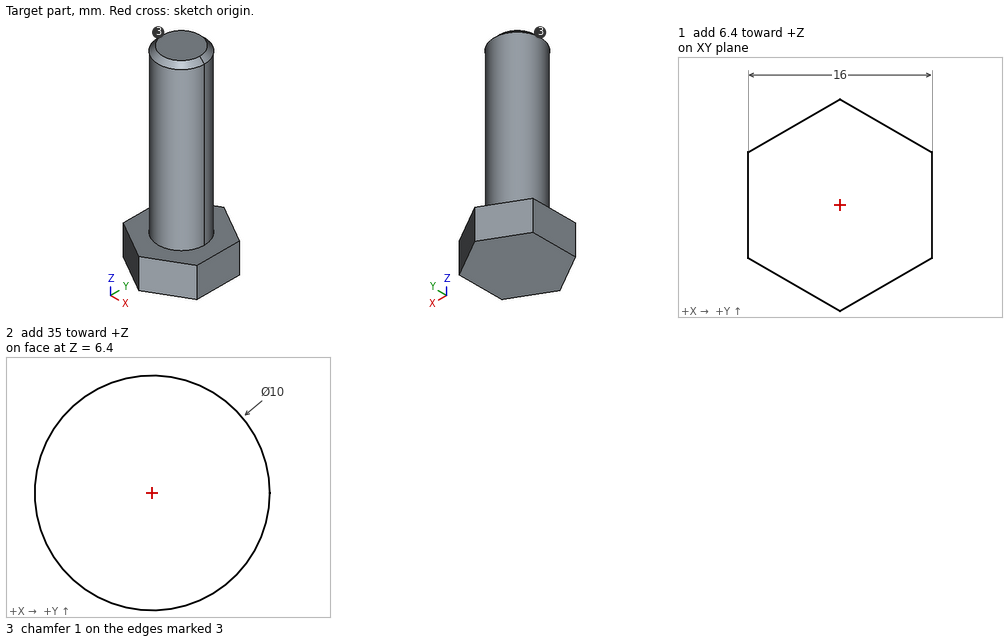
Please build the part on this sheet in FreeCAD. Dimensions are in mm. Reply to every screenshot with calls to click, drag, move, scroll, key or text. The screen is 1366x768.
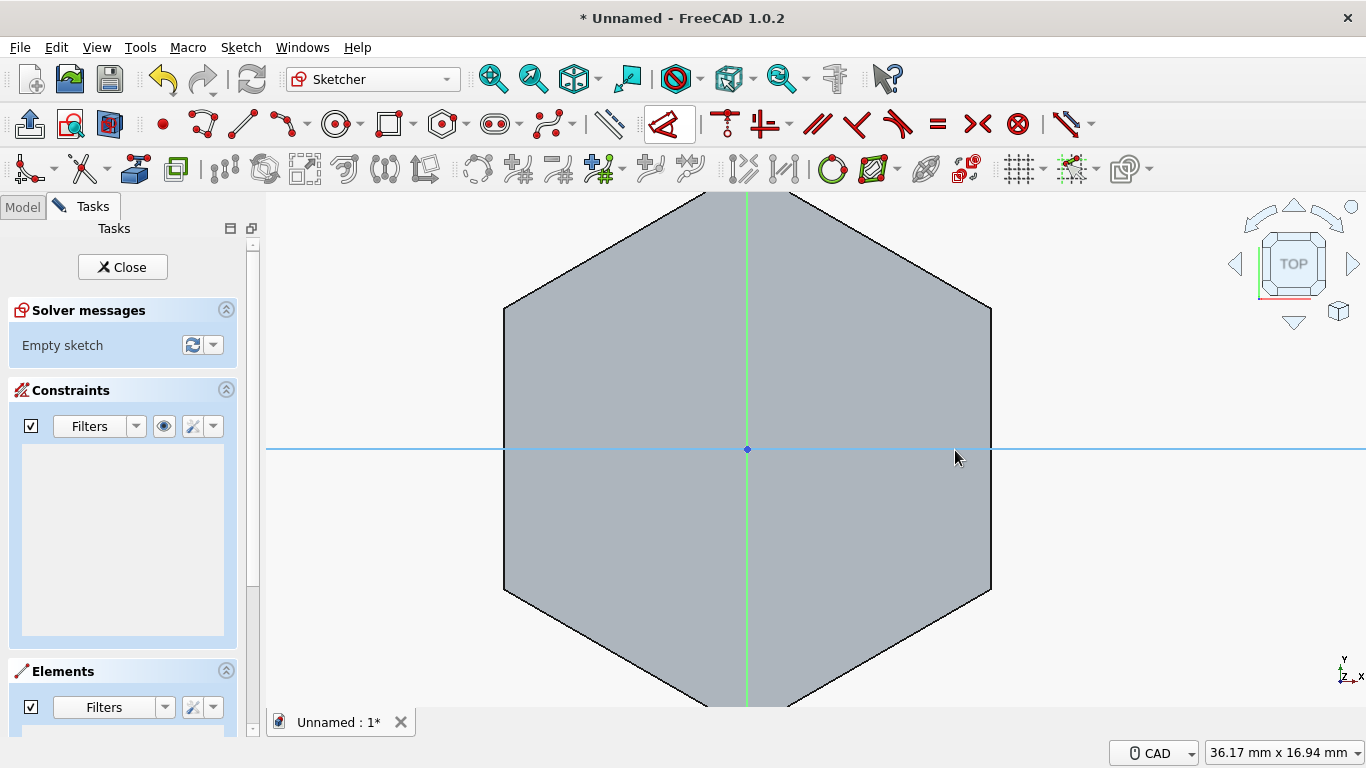
click(336, 124)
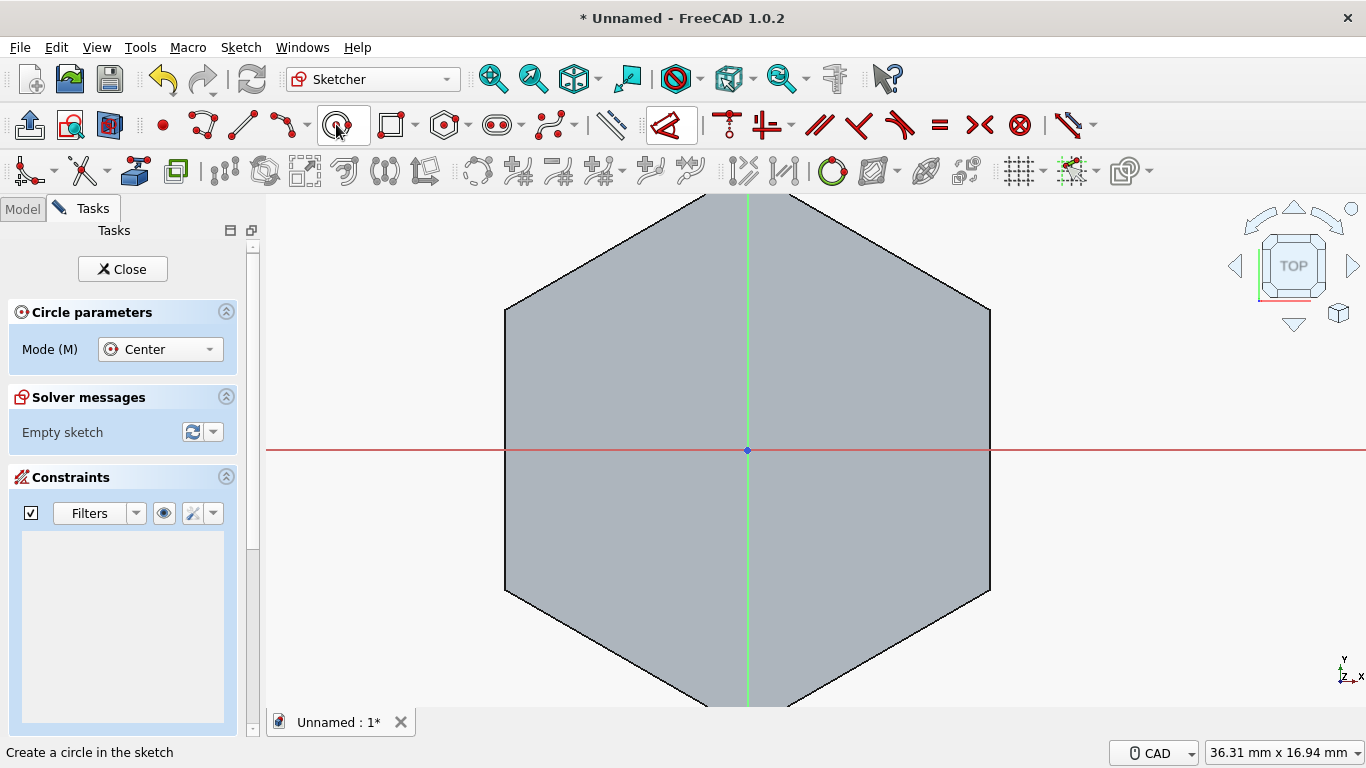
click(748, 450)
click(855, 343)
key(Escape)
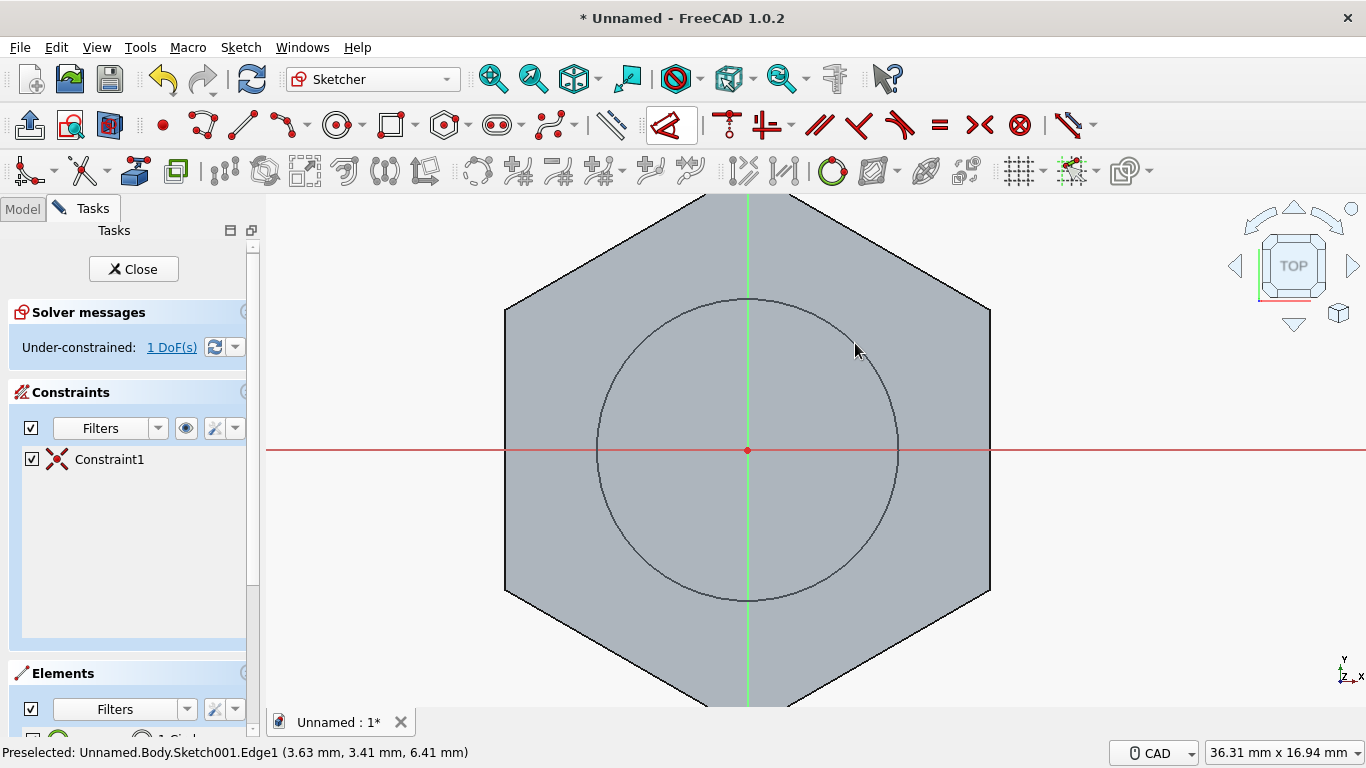
click(666, 126)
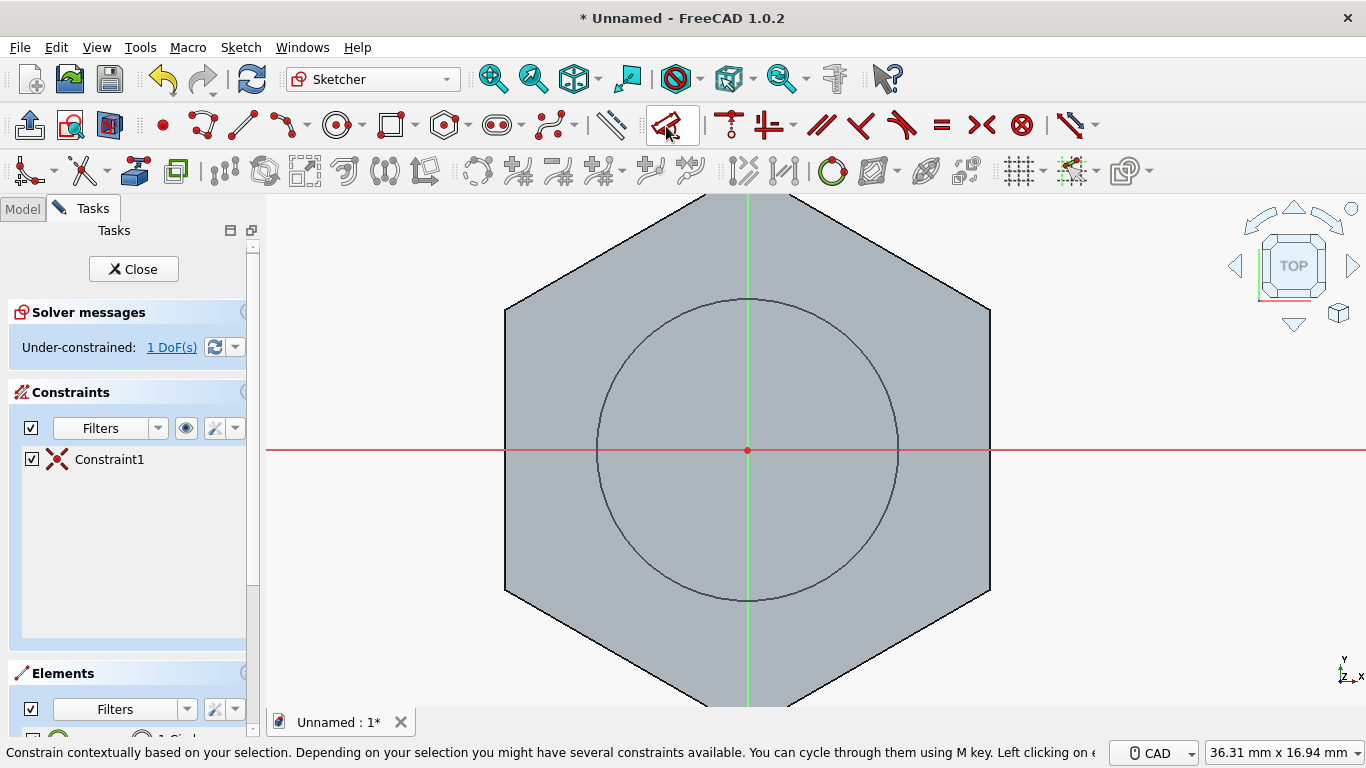
click(854, 343)
click(877, 320)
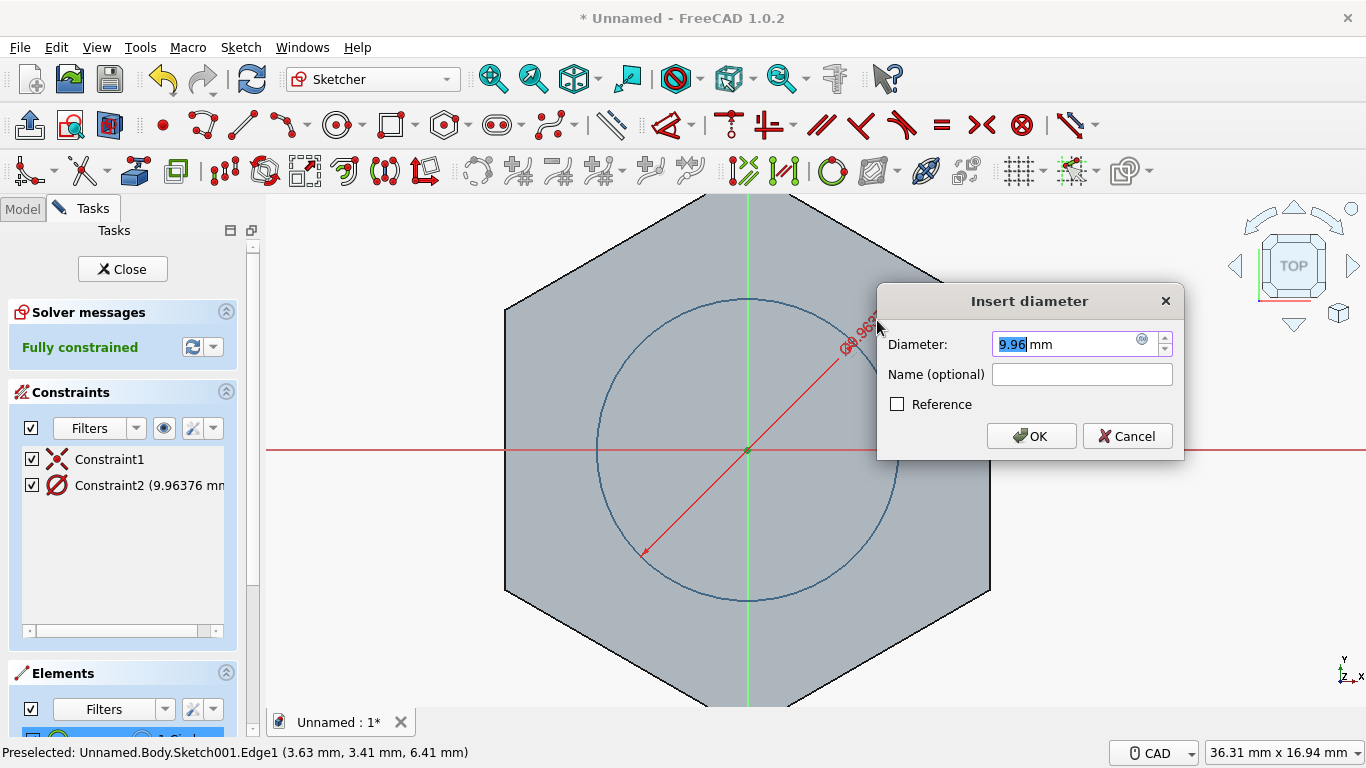
text(10)
key(Return)
key(Escape)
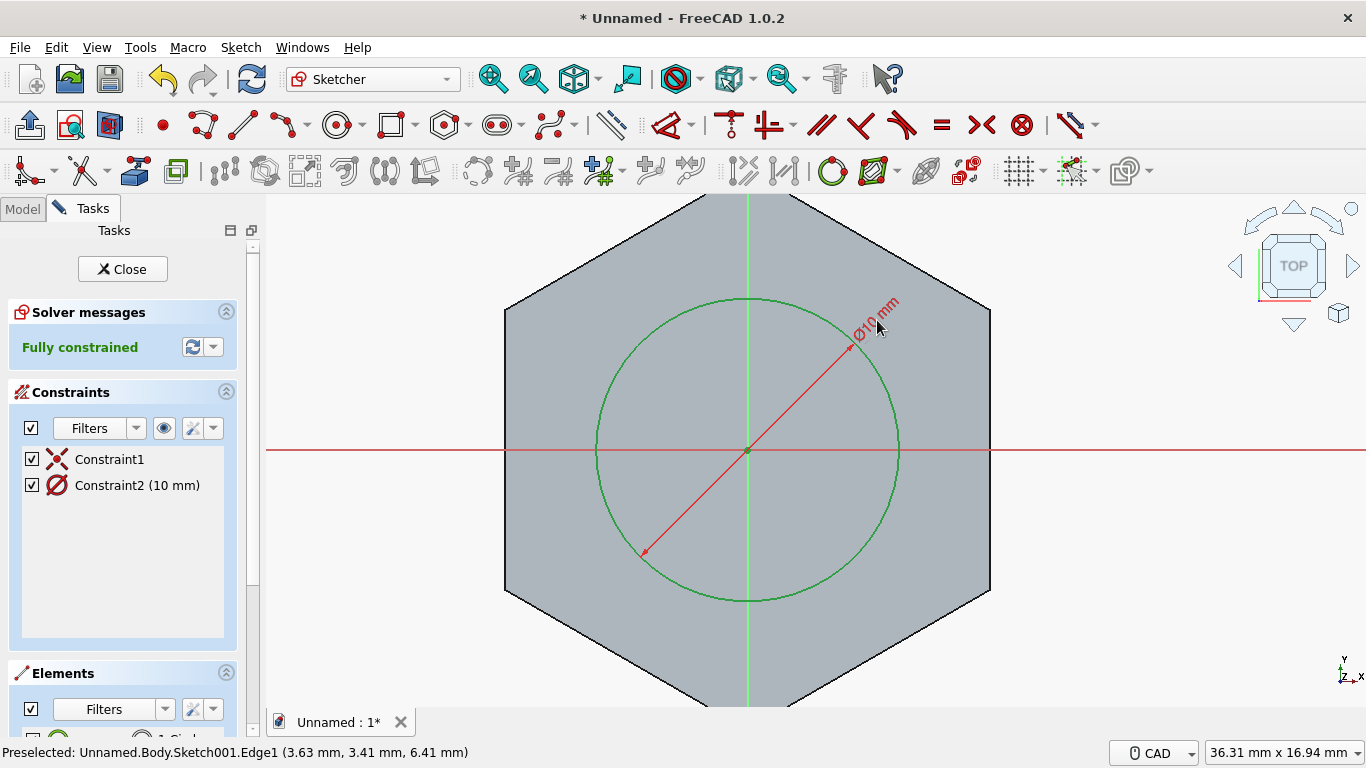
click(123, 269)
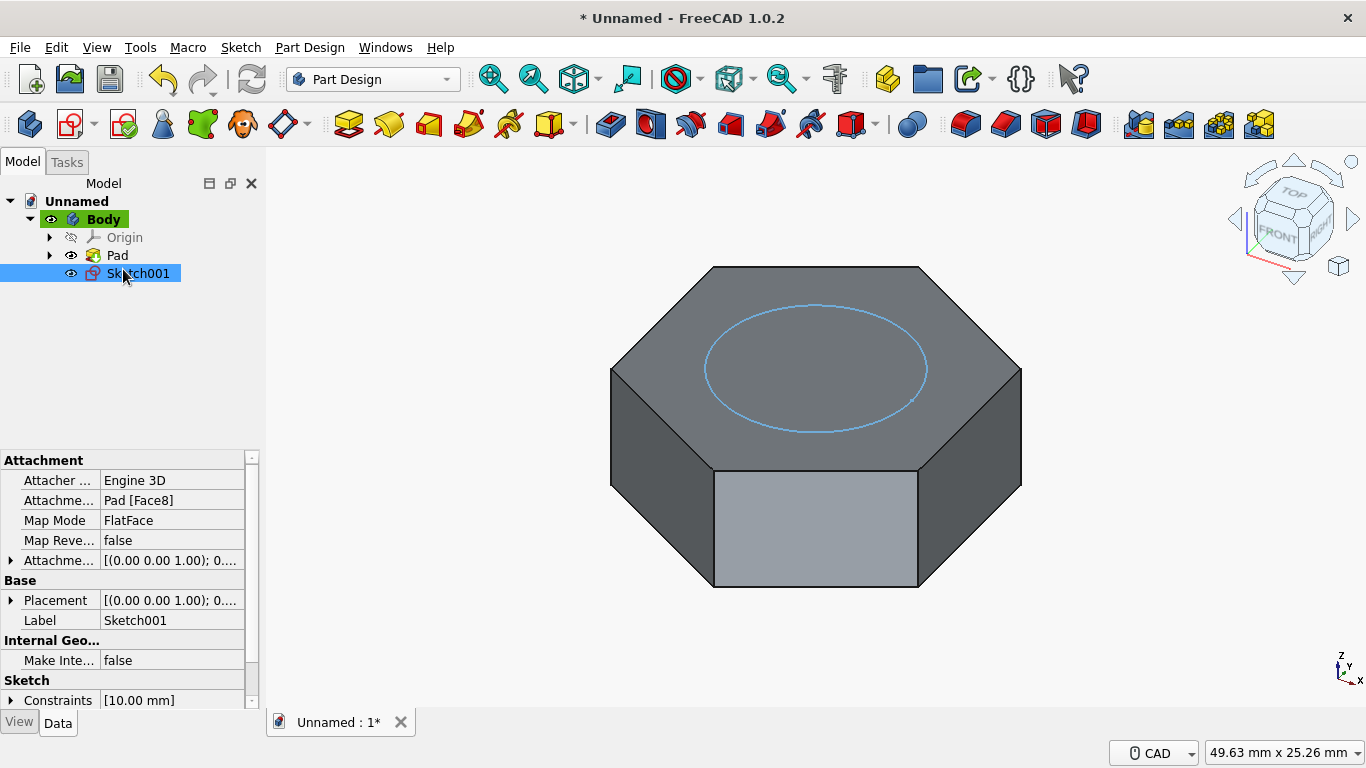
click(350, 124)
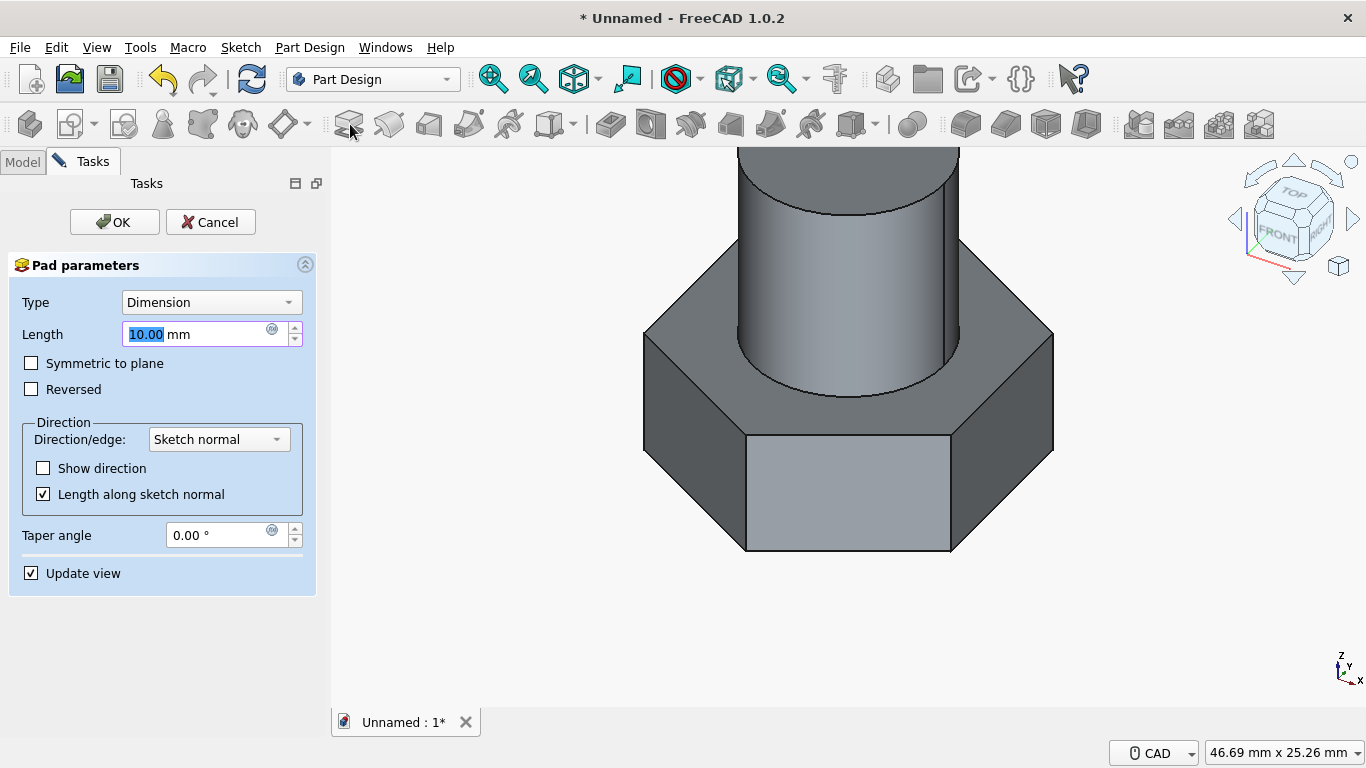
text(35)
key(Tab)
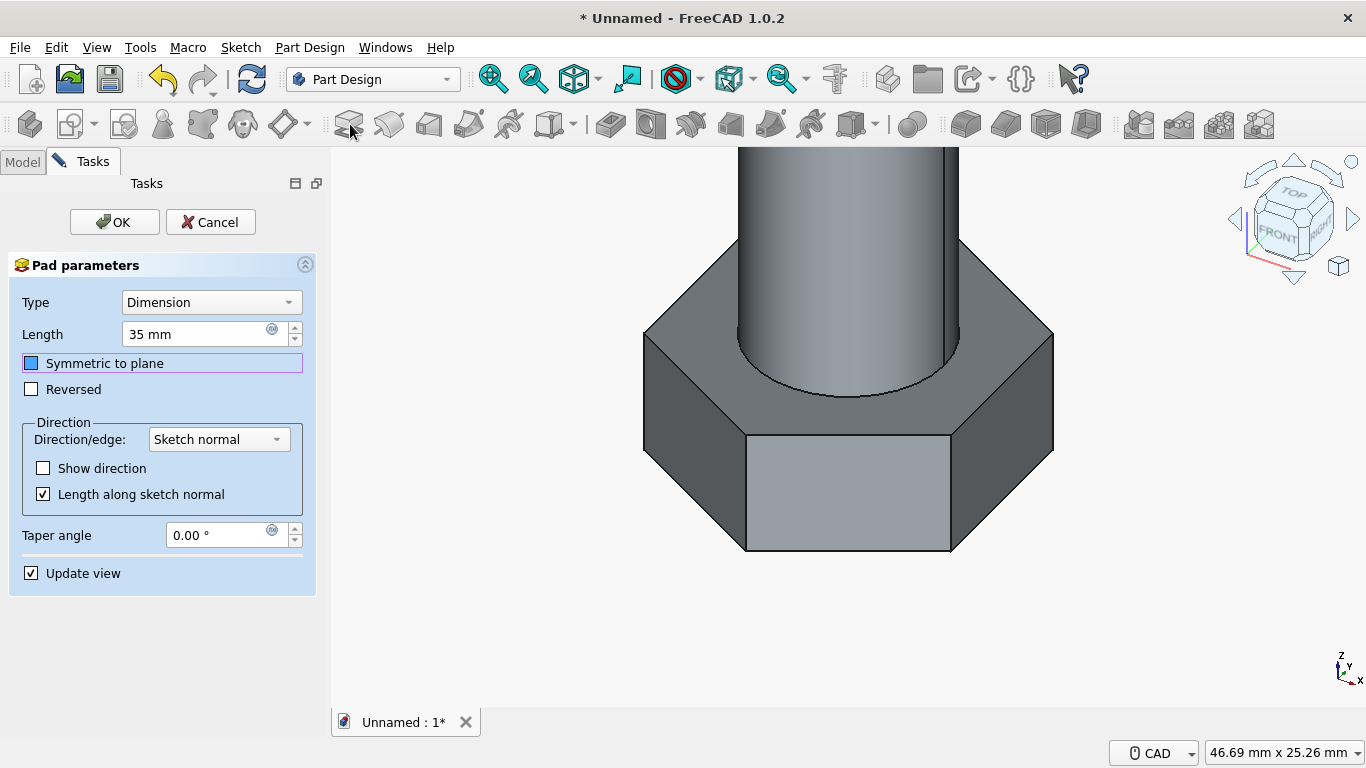
click(115, 222)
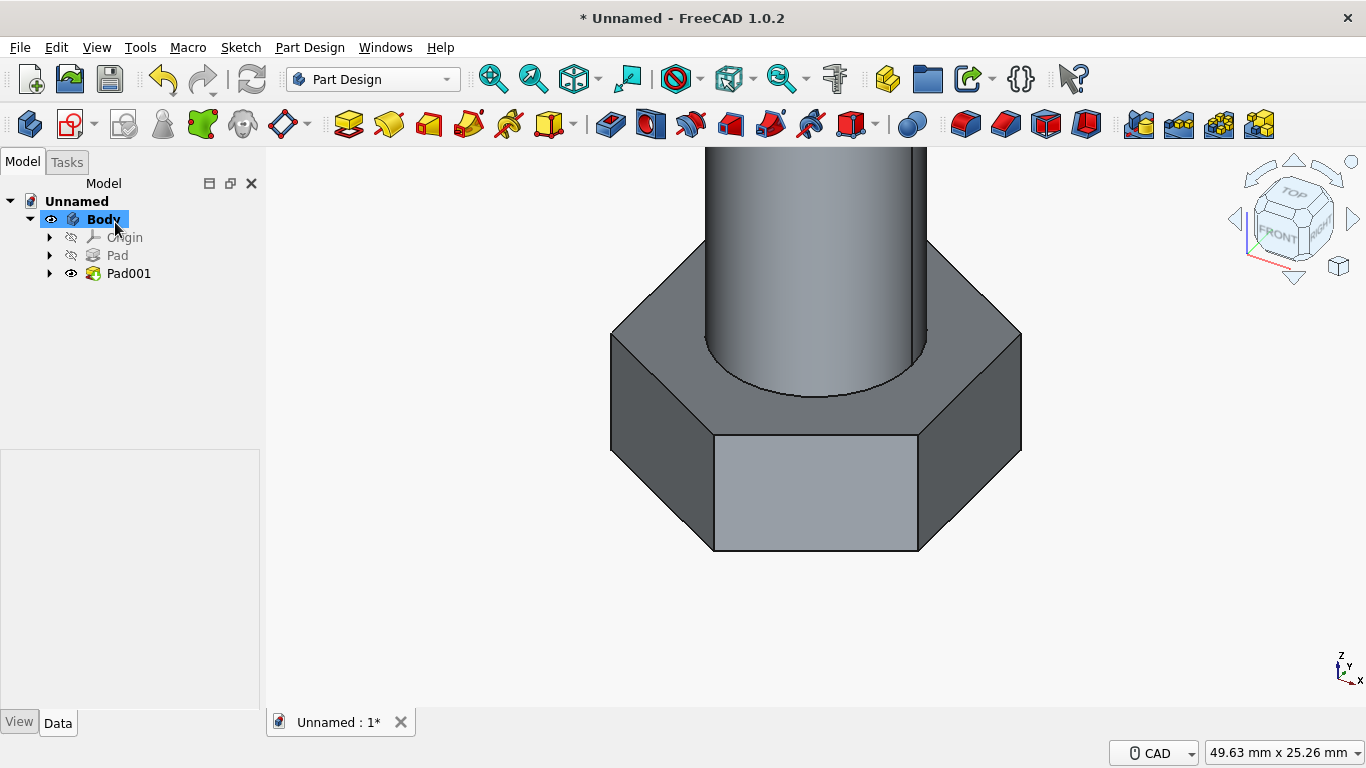
click(494, 80)